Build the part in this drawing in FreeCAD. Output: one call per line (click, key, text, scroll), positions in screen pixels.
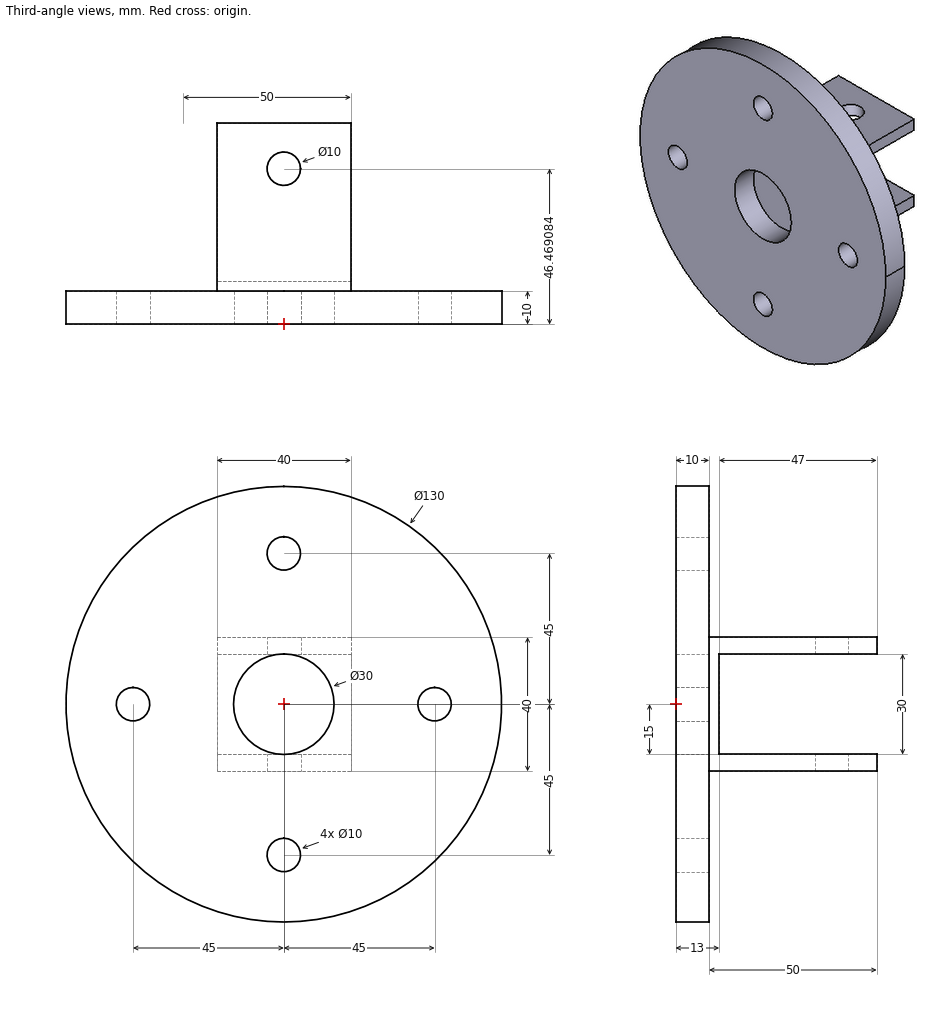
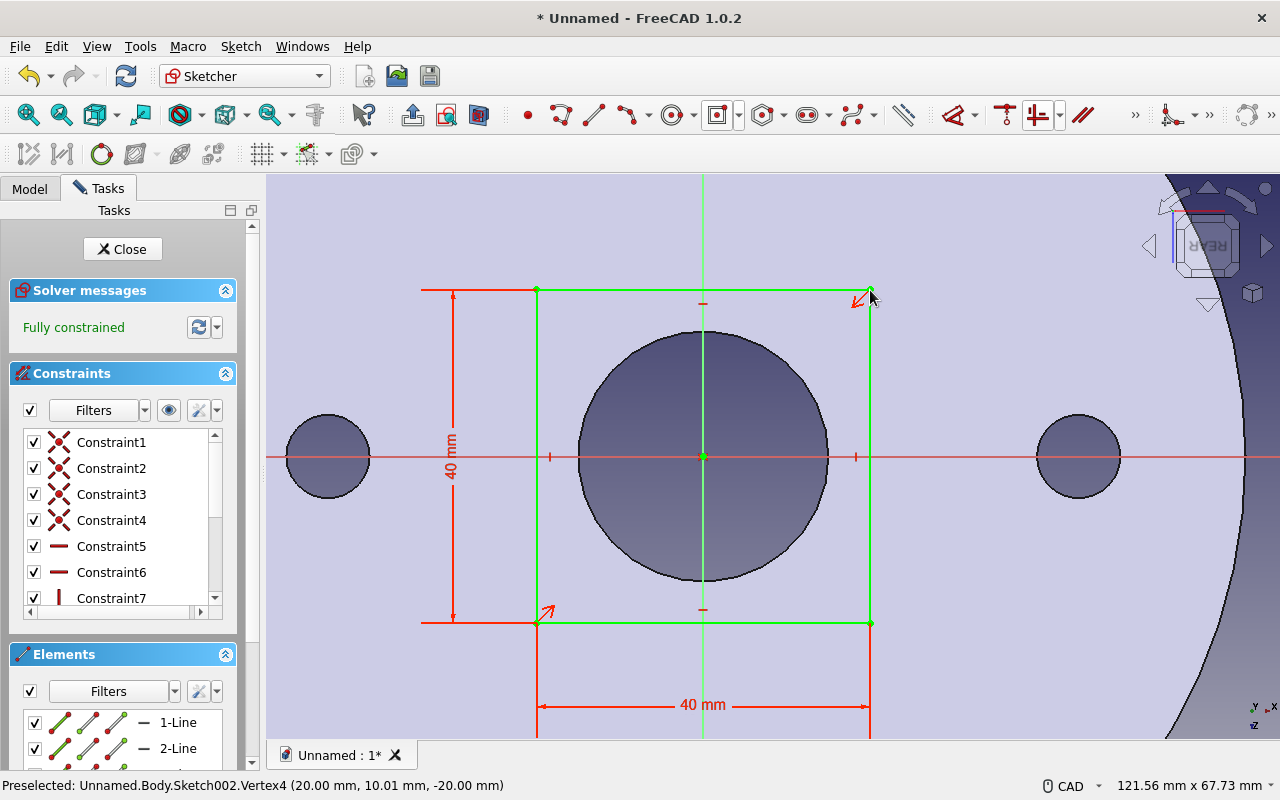
click(123, 249)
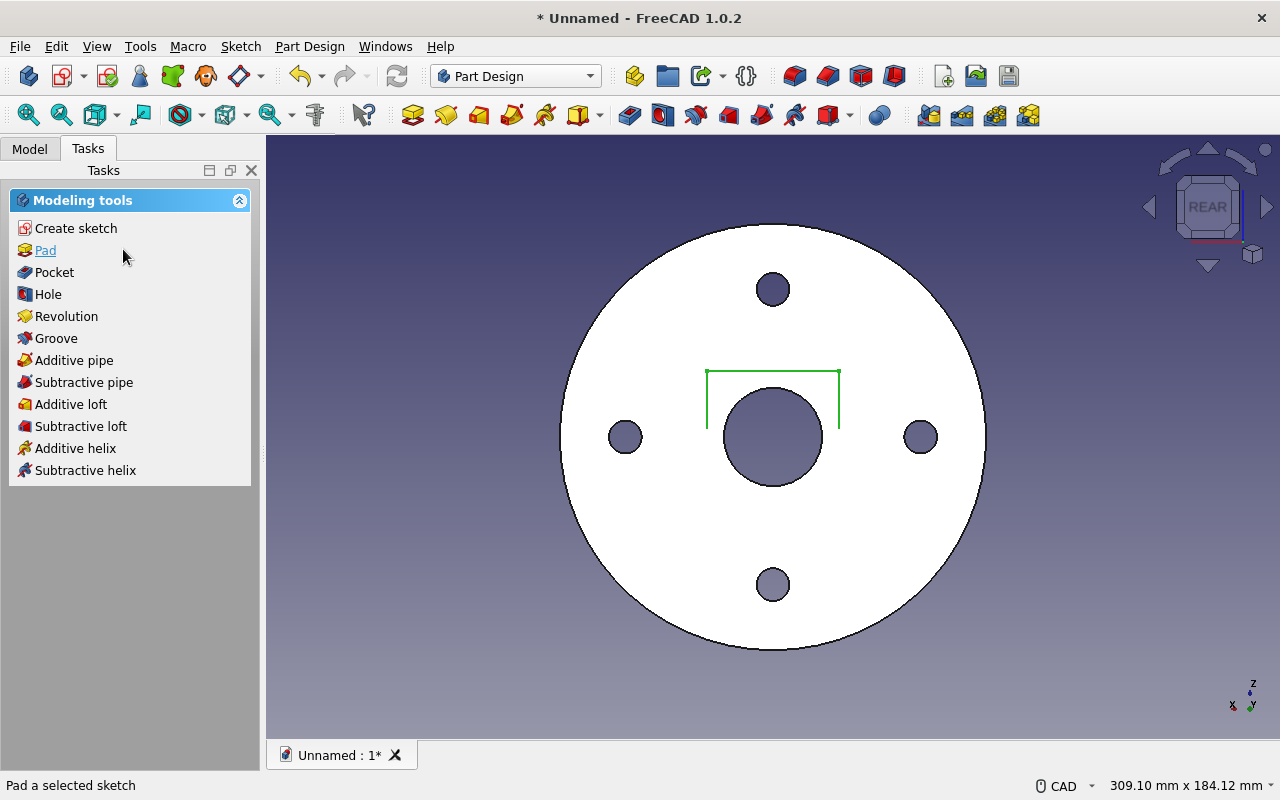
click(413, 116)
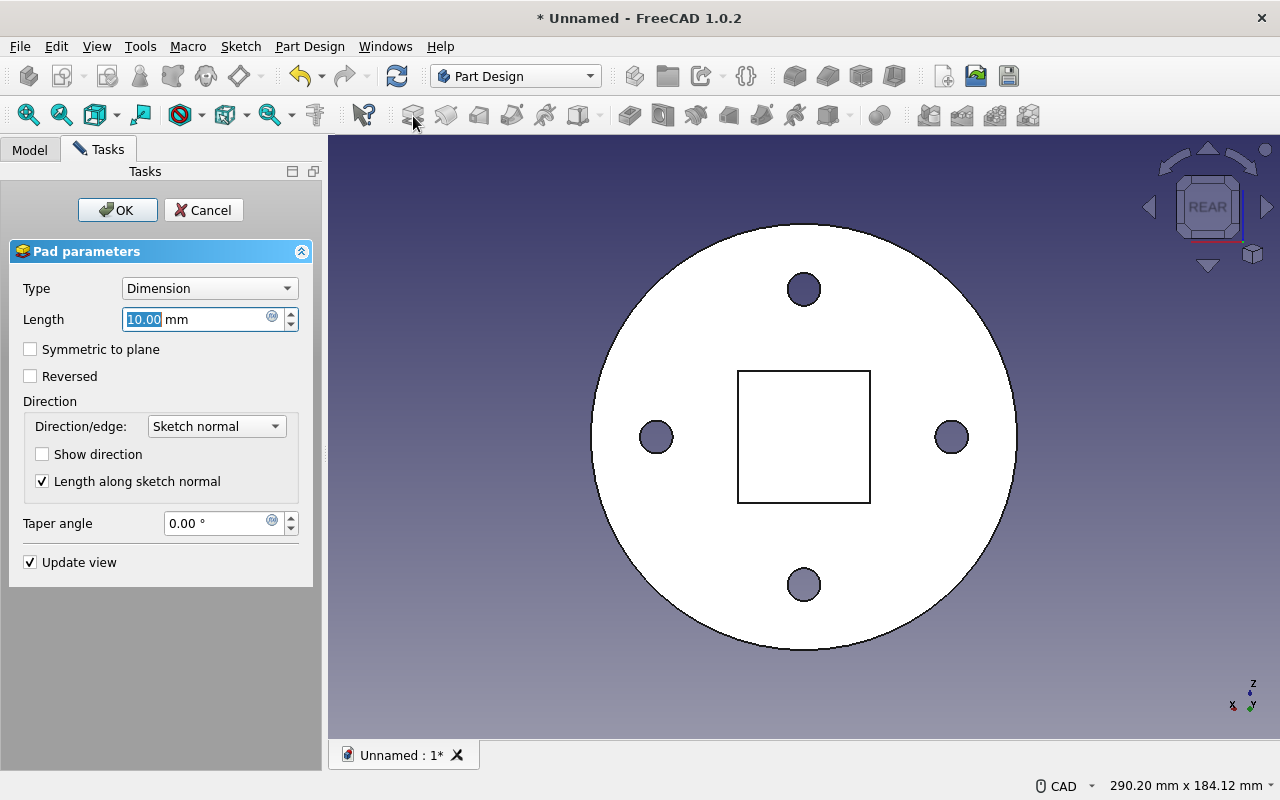
text(50)
key(Tab)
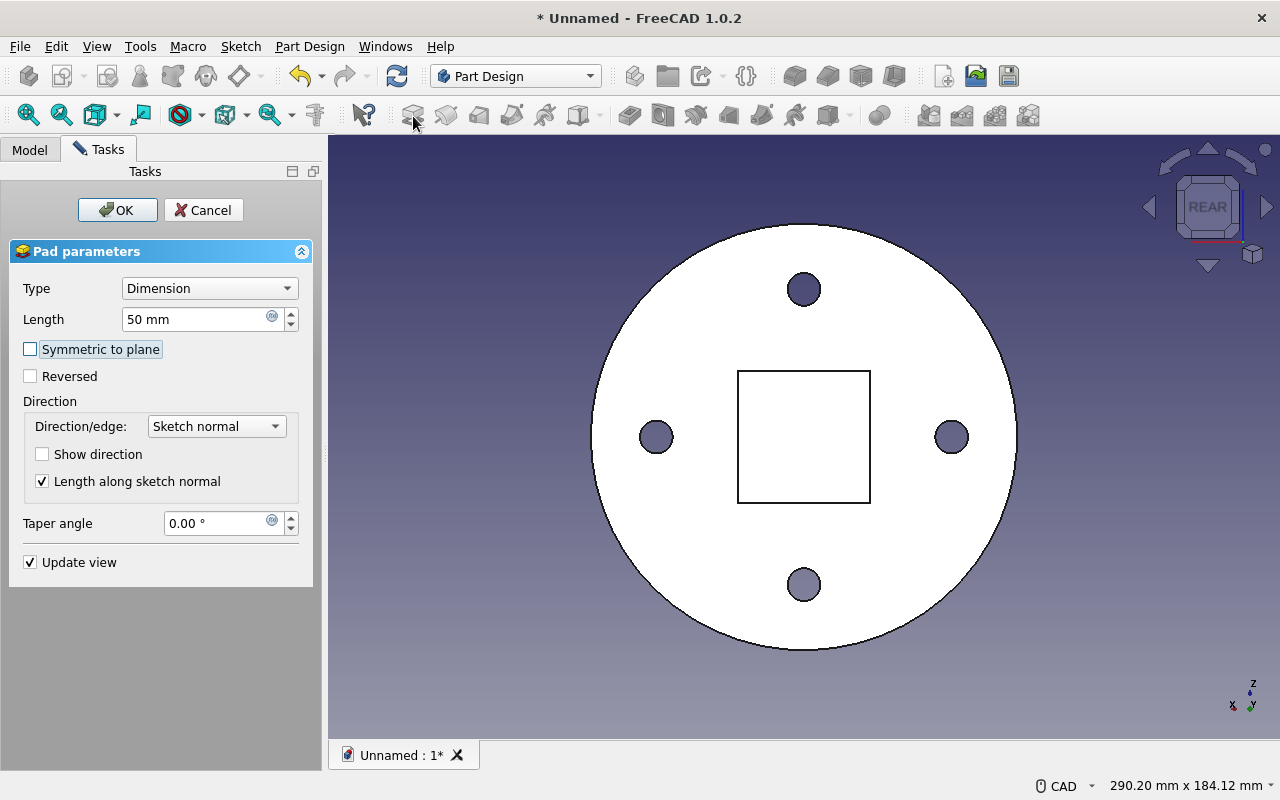
click(118, 210)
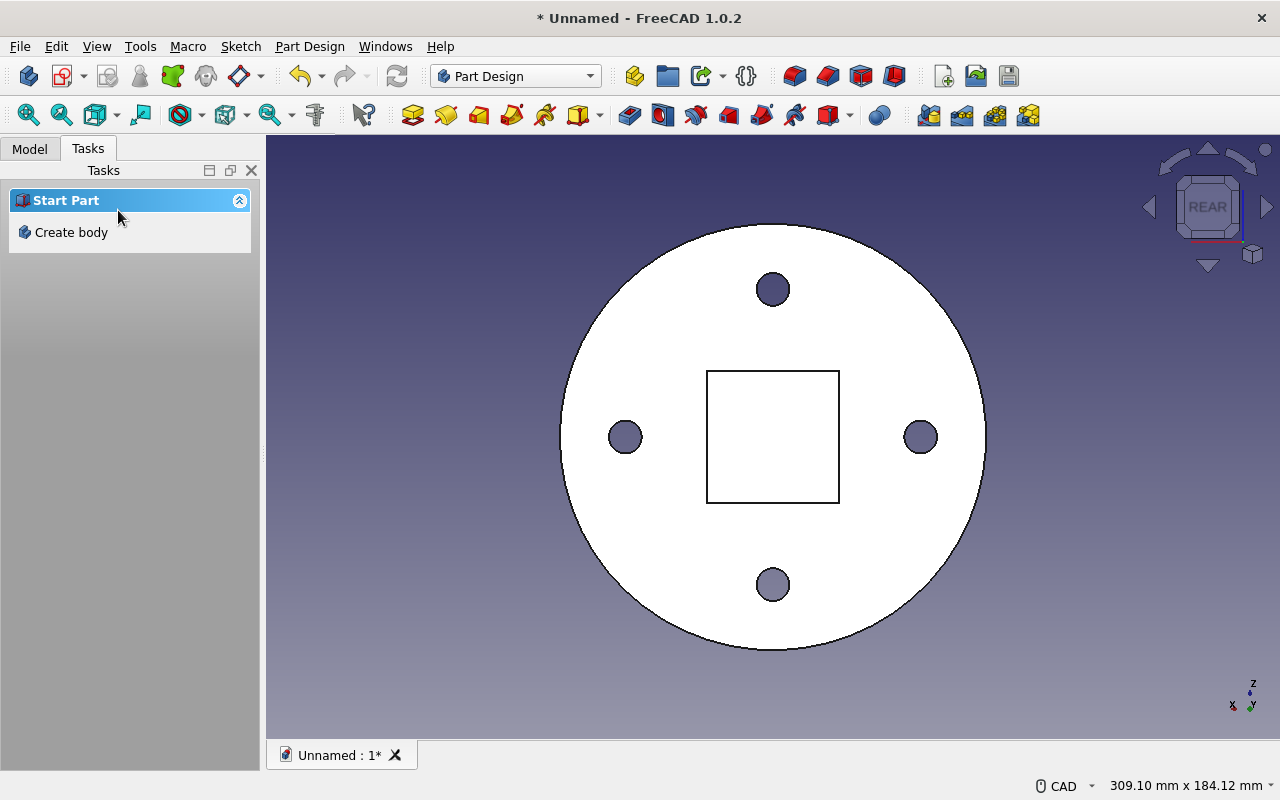
key(0)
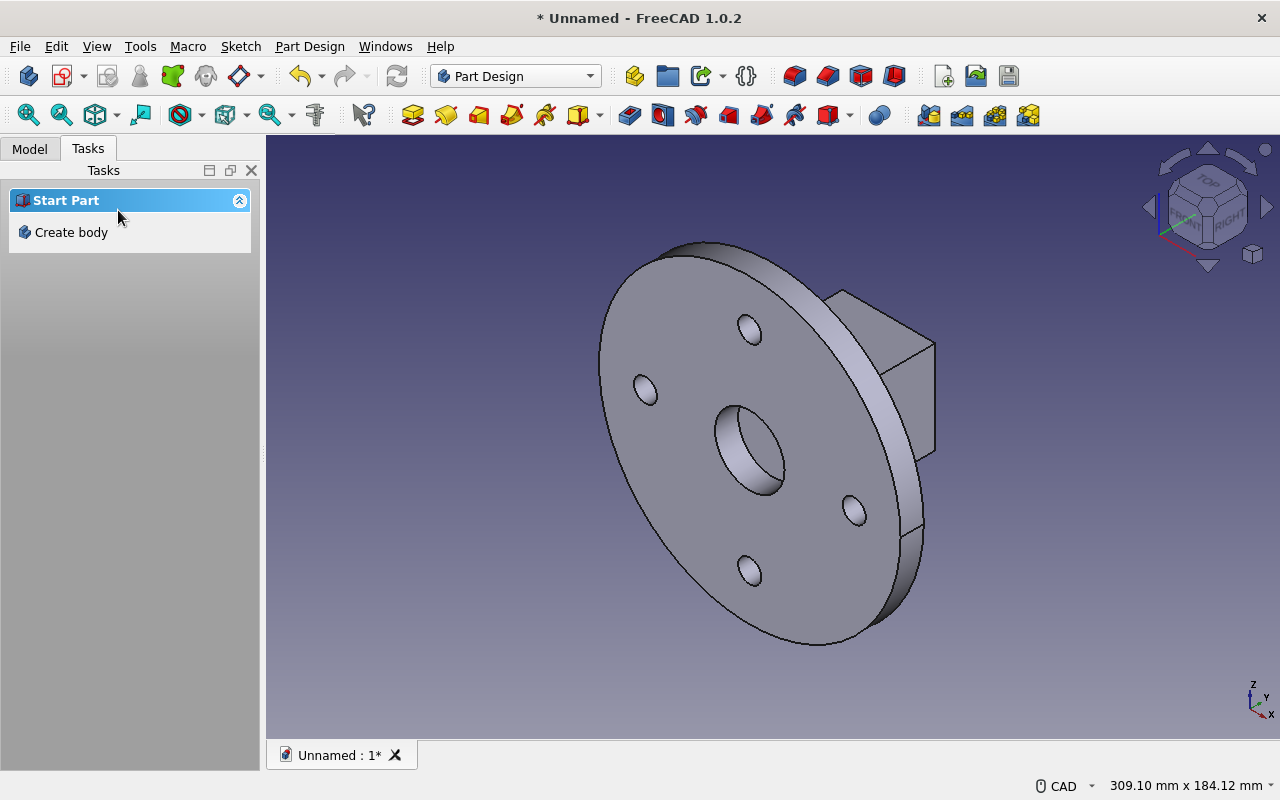
key(v)
key(f)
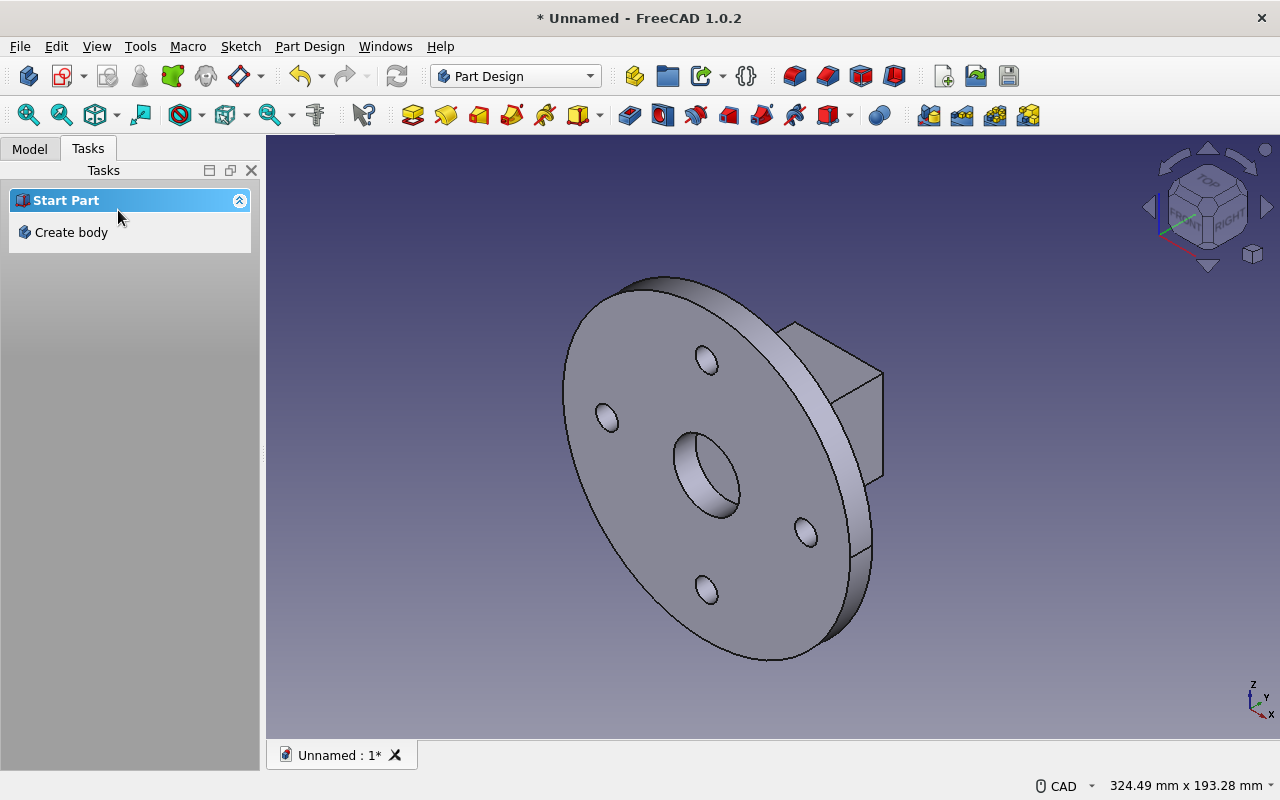
key(3)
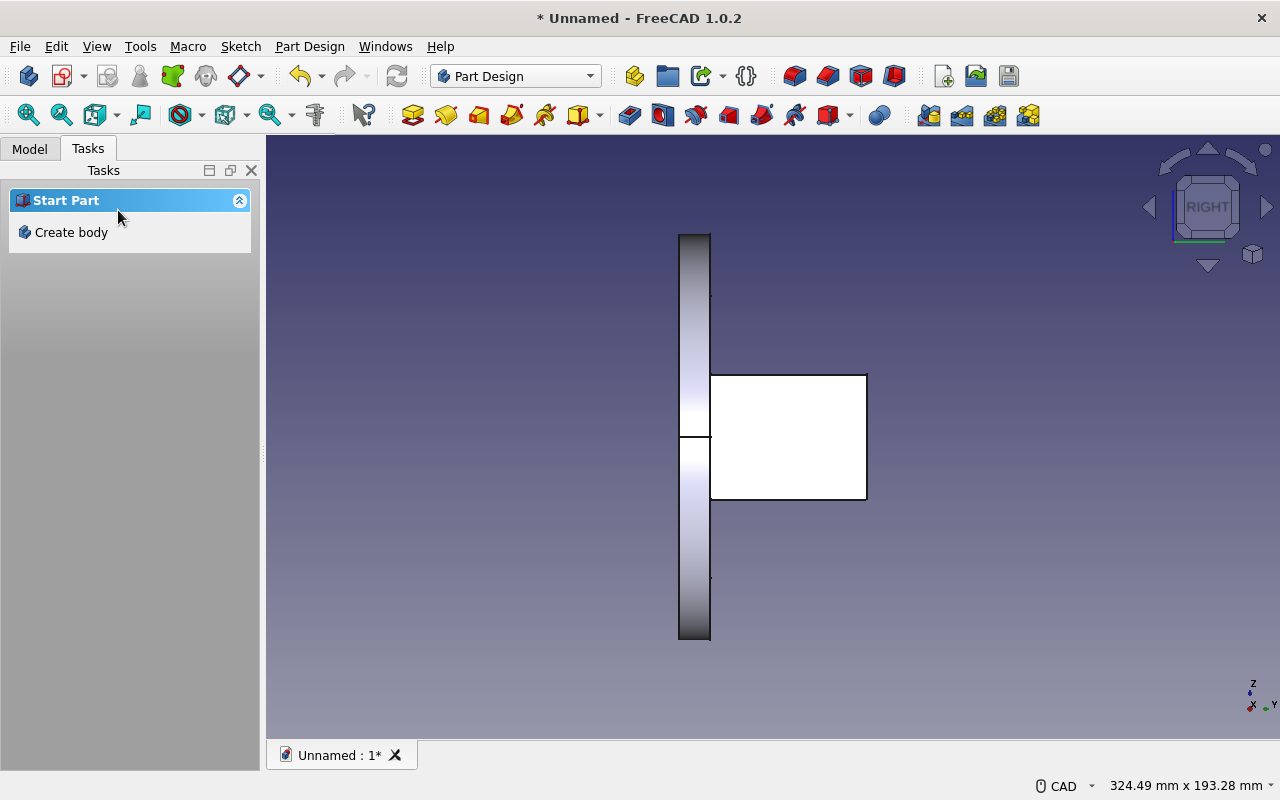
click(789, 436)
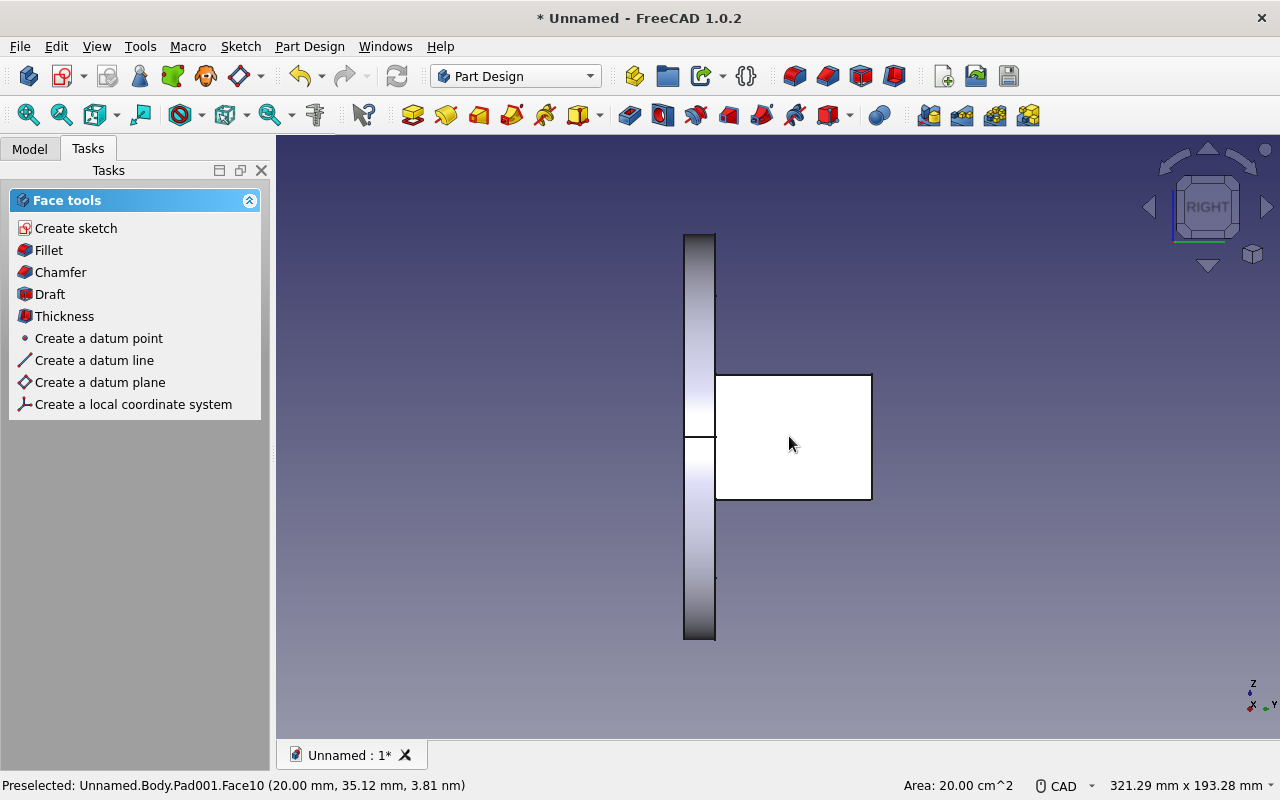
click(62, 76)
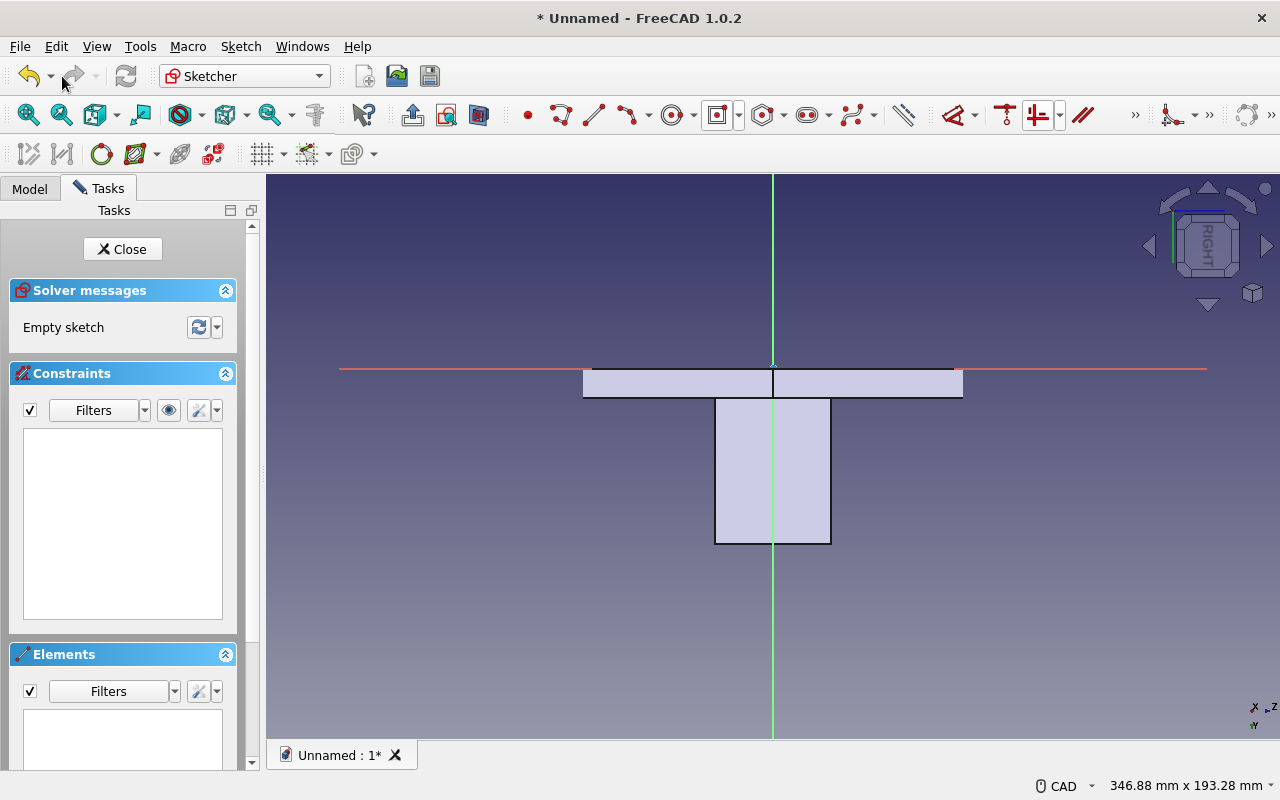
click(479, 116)